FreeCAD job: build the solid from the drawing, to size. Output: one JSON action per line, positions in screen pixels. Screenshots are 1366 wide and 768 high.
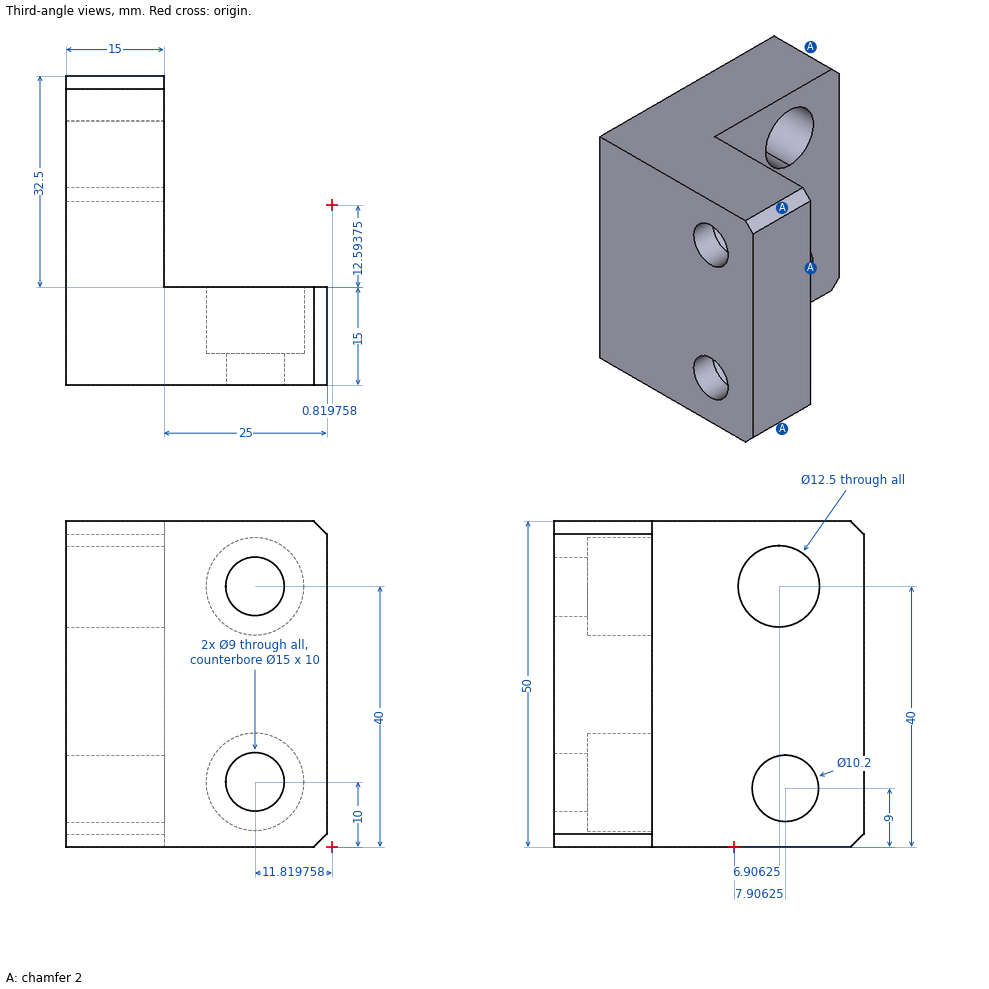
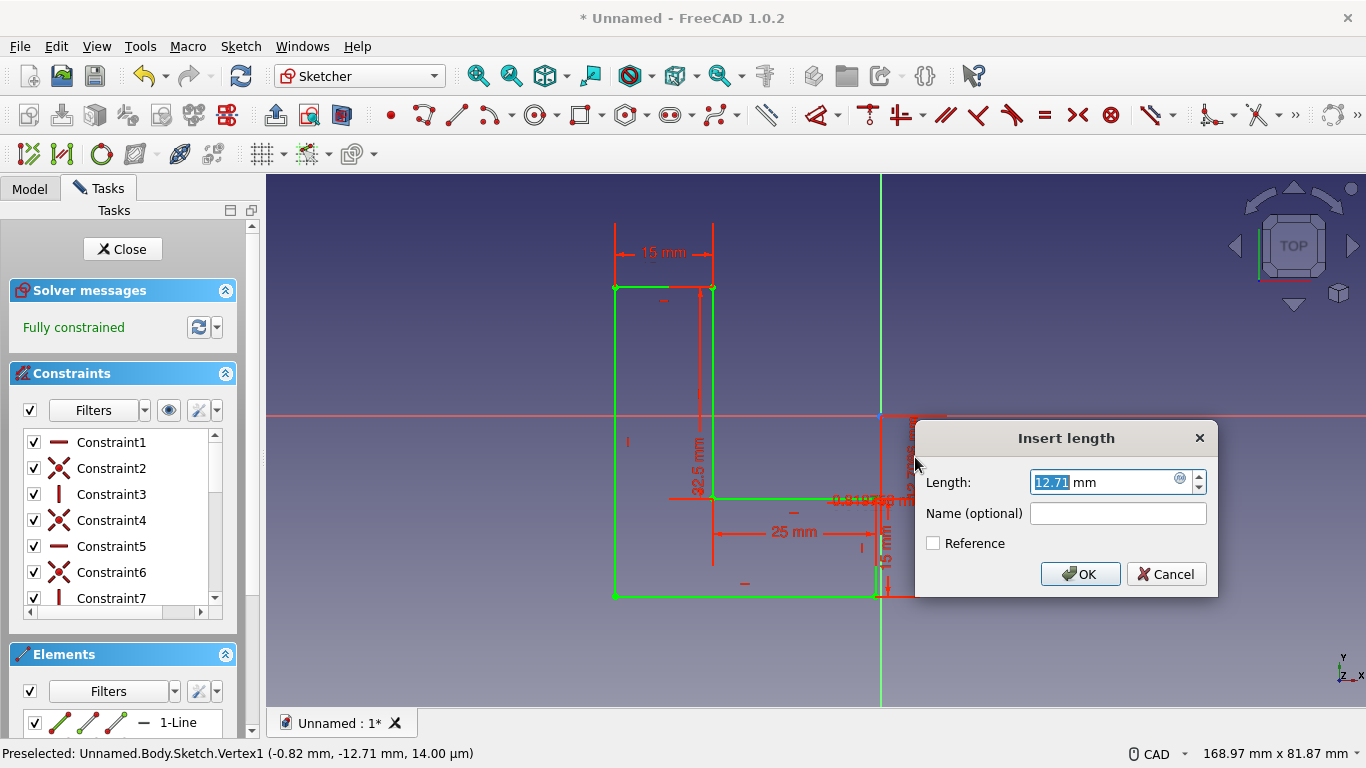
{"action": "type", "text": "12.59375"}
{"action": "key", "text": "Return"}
{"action": "key", "text": "Escape"}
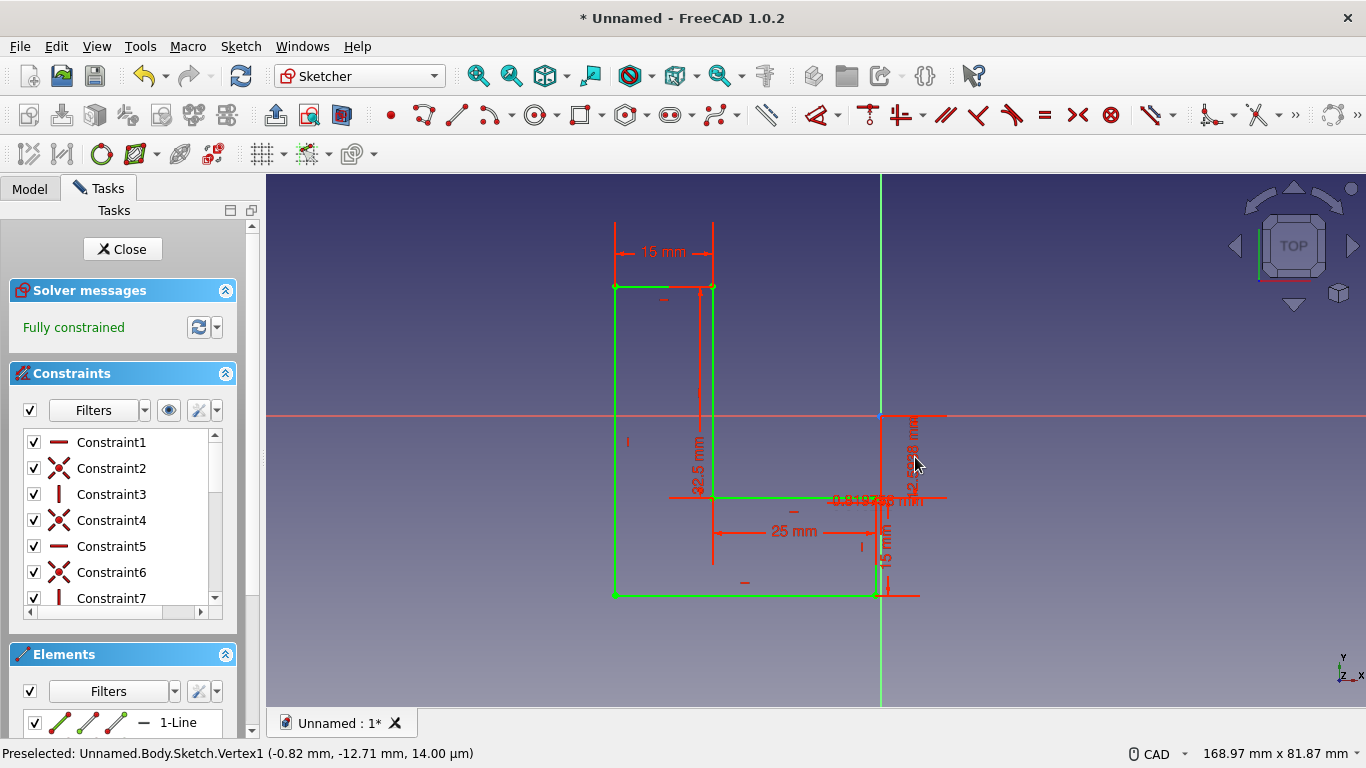
{"action": "left_click", "coordinate": [123, 249]}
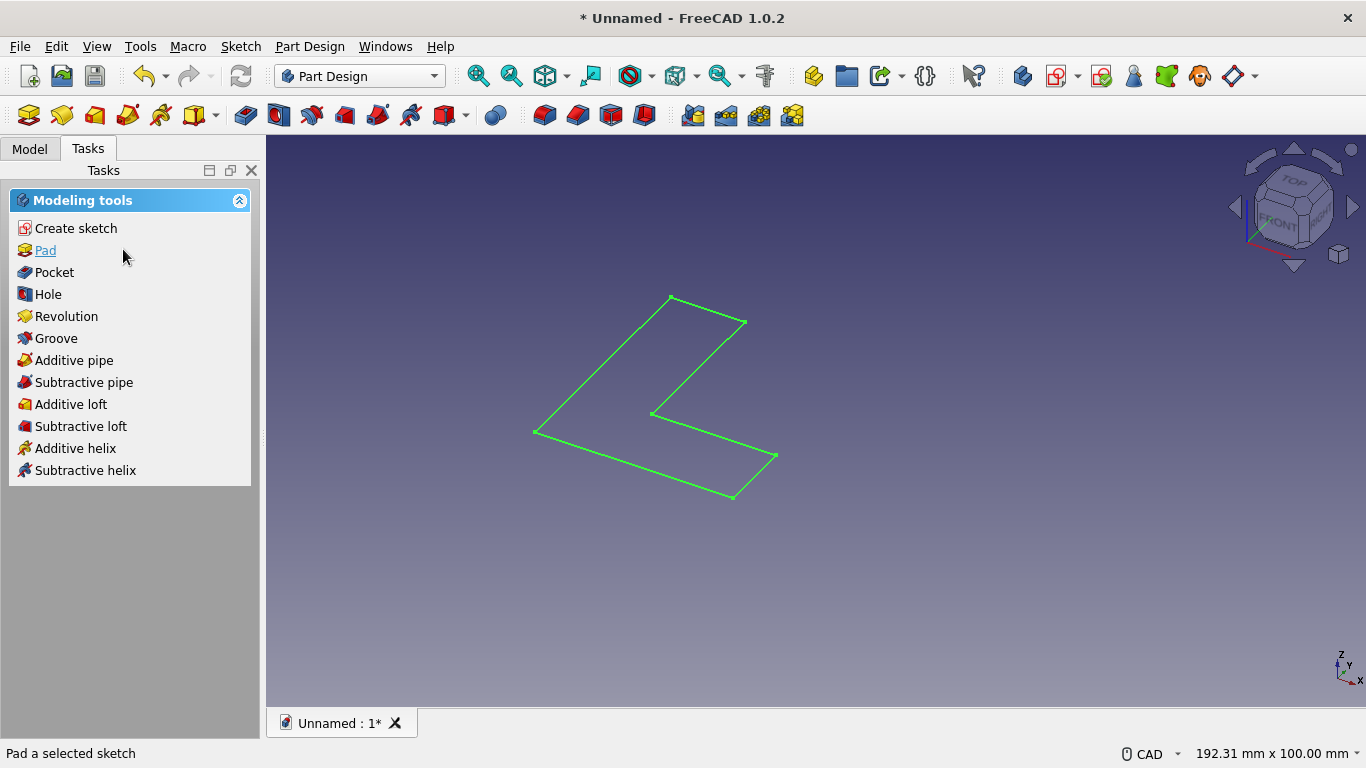
{"action": "left_click", "coordinate": [29, 116]}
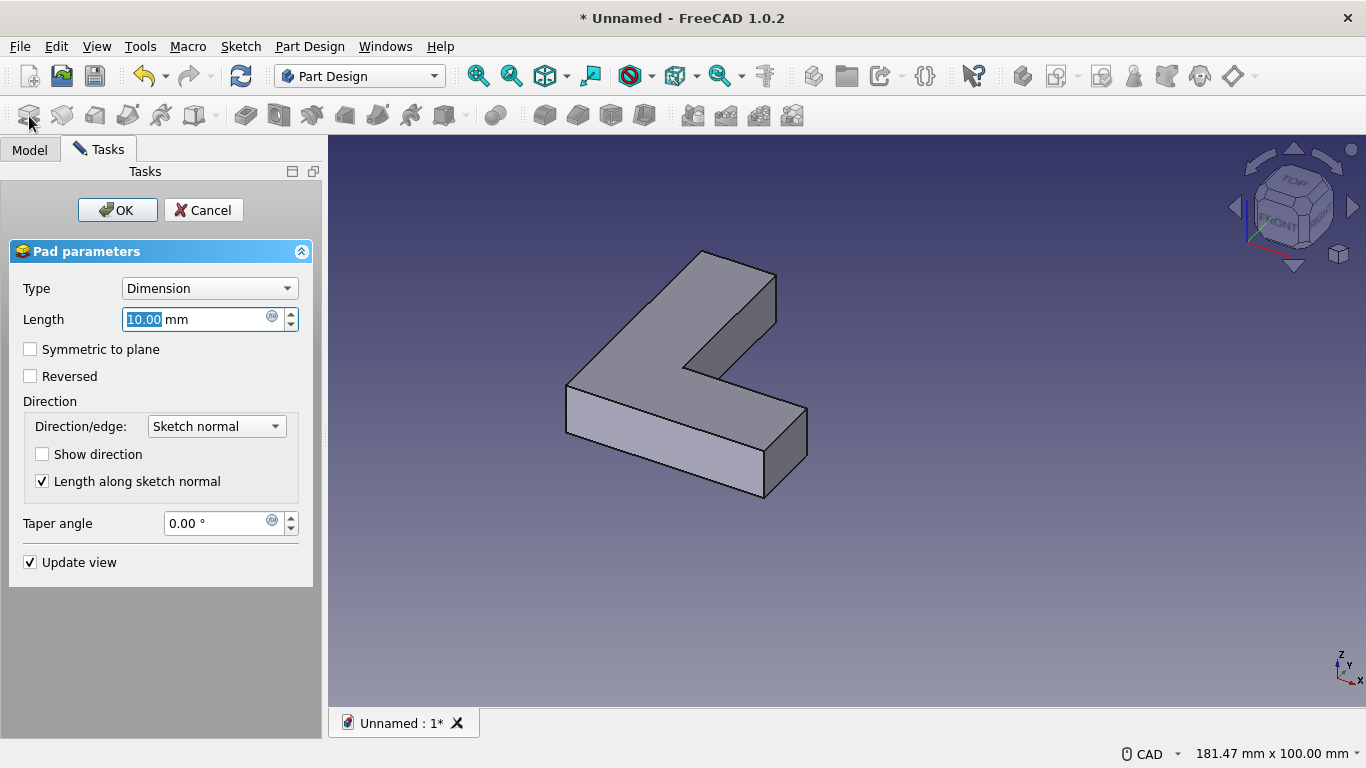
{"action": "type", "text": "50"}
{"action": "key", "text": "Tab"}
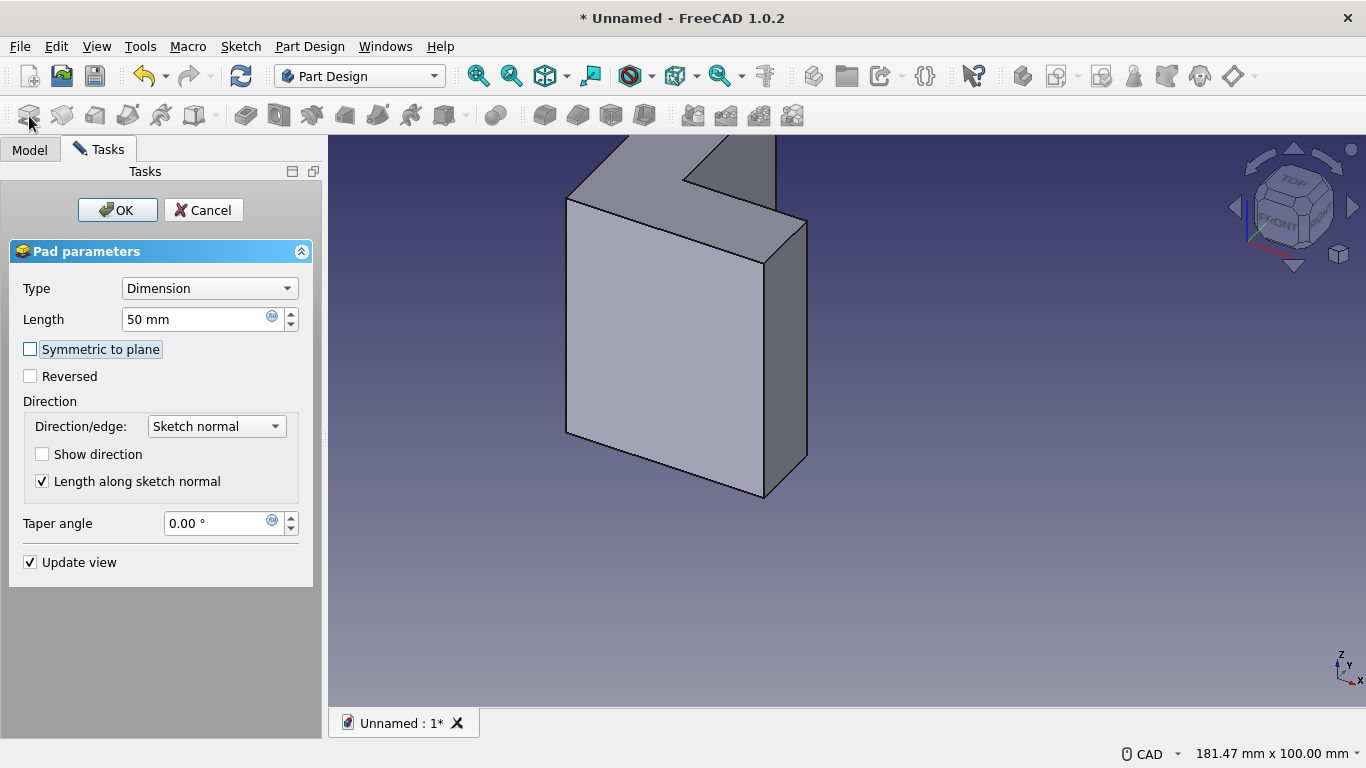
{"action": "left_click", "coordinate": [118, 210]}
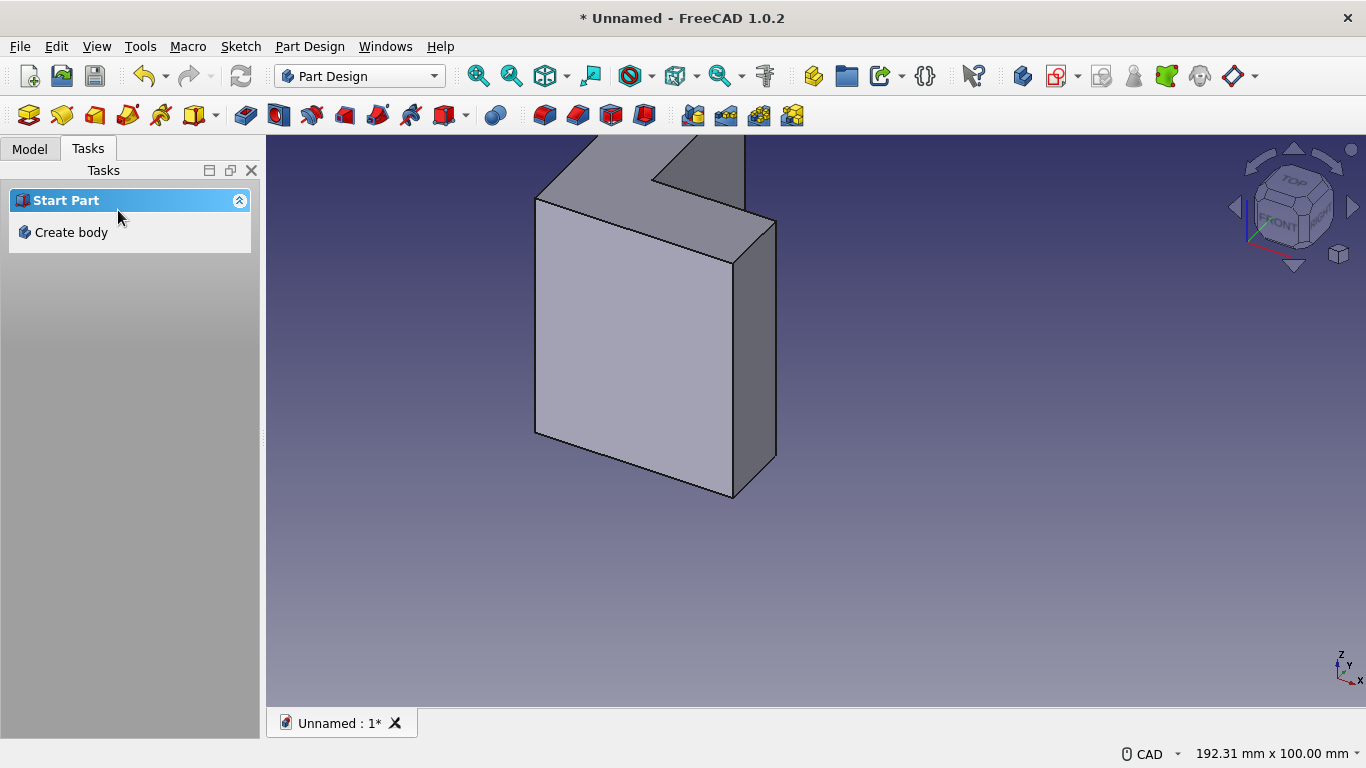
{"action": "left_click", "coordinate": [479, 76]}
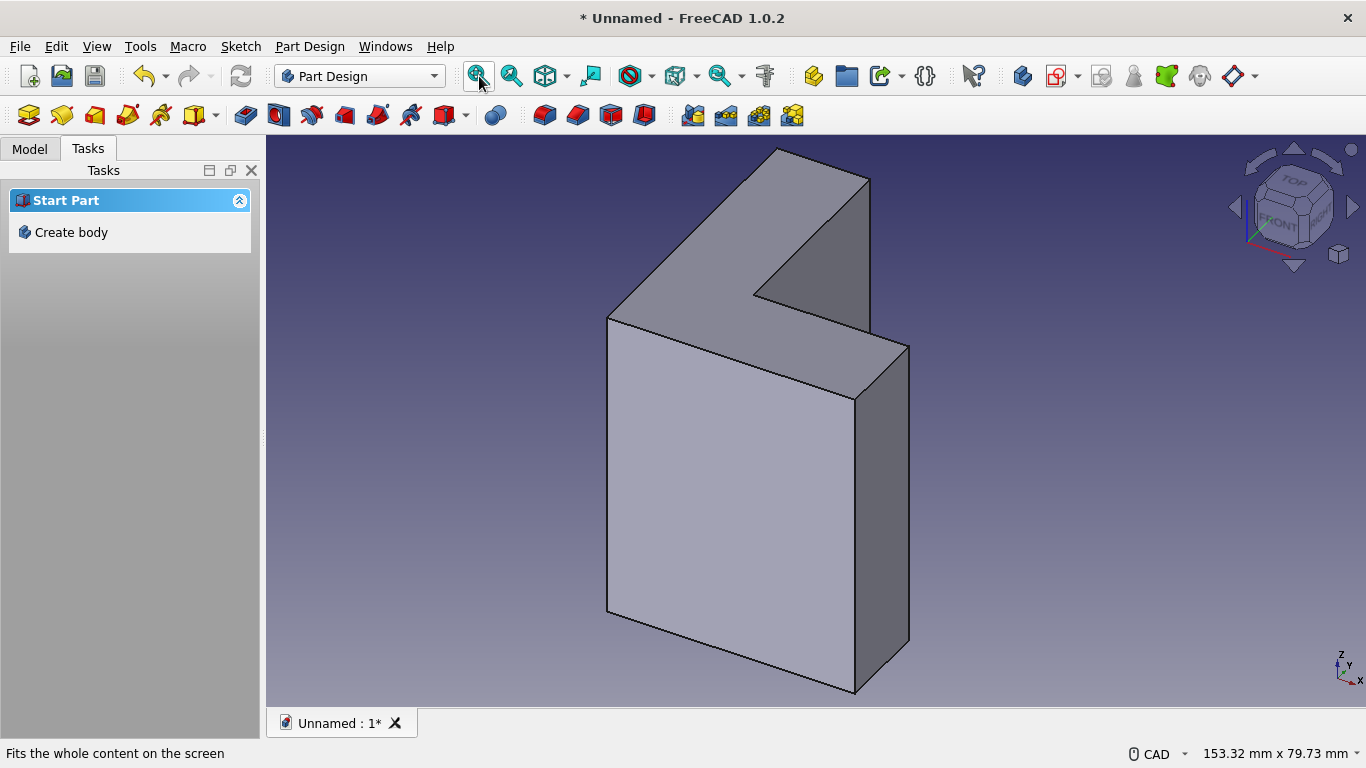
{"action": "left_click", "coordinate": [882, 372]}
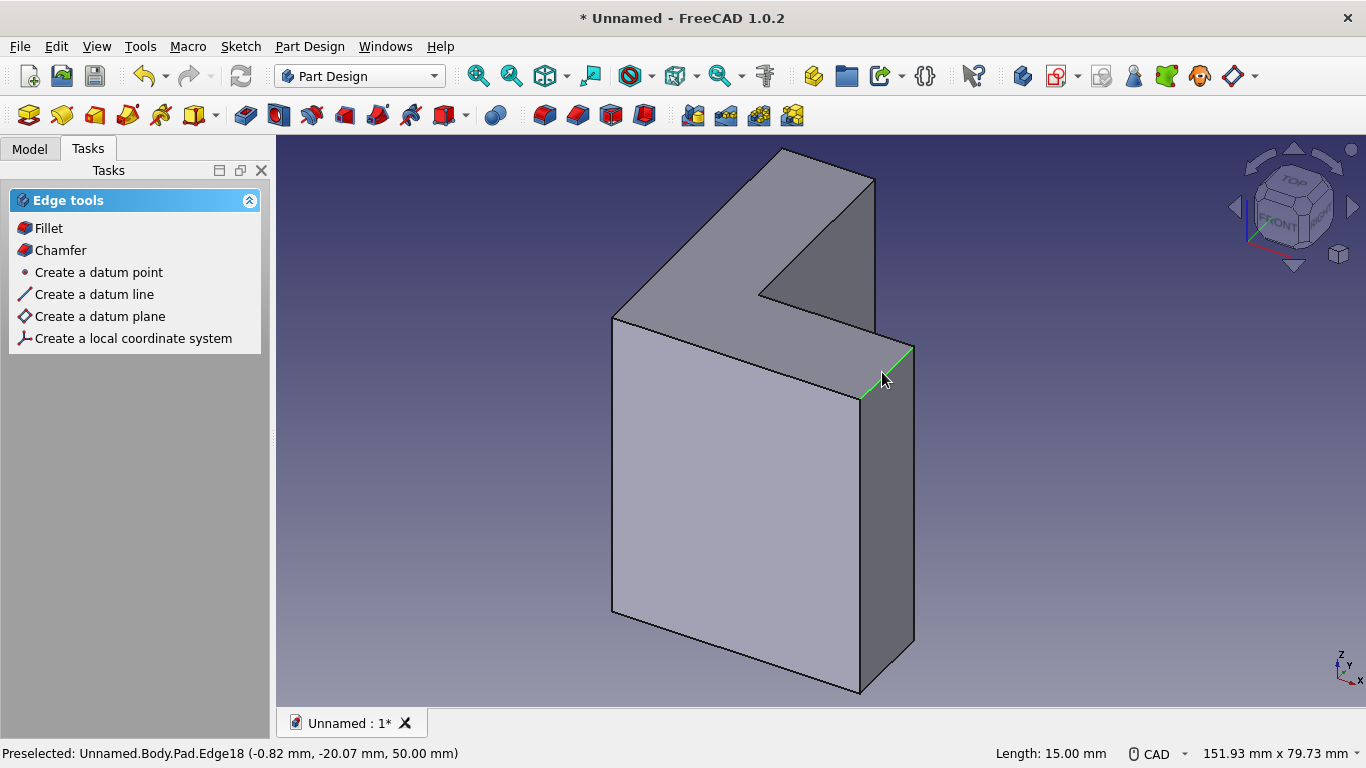
{"action": "key", "text": "0"}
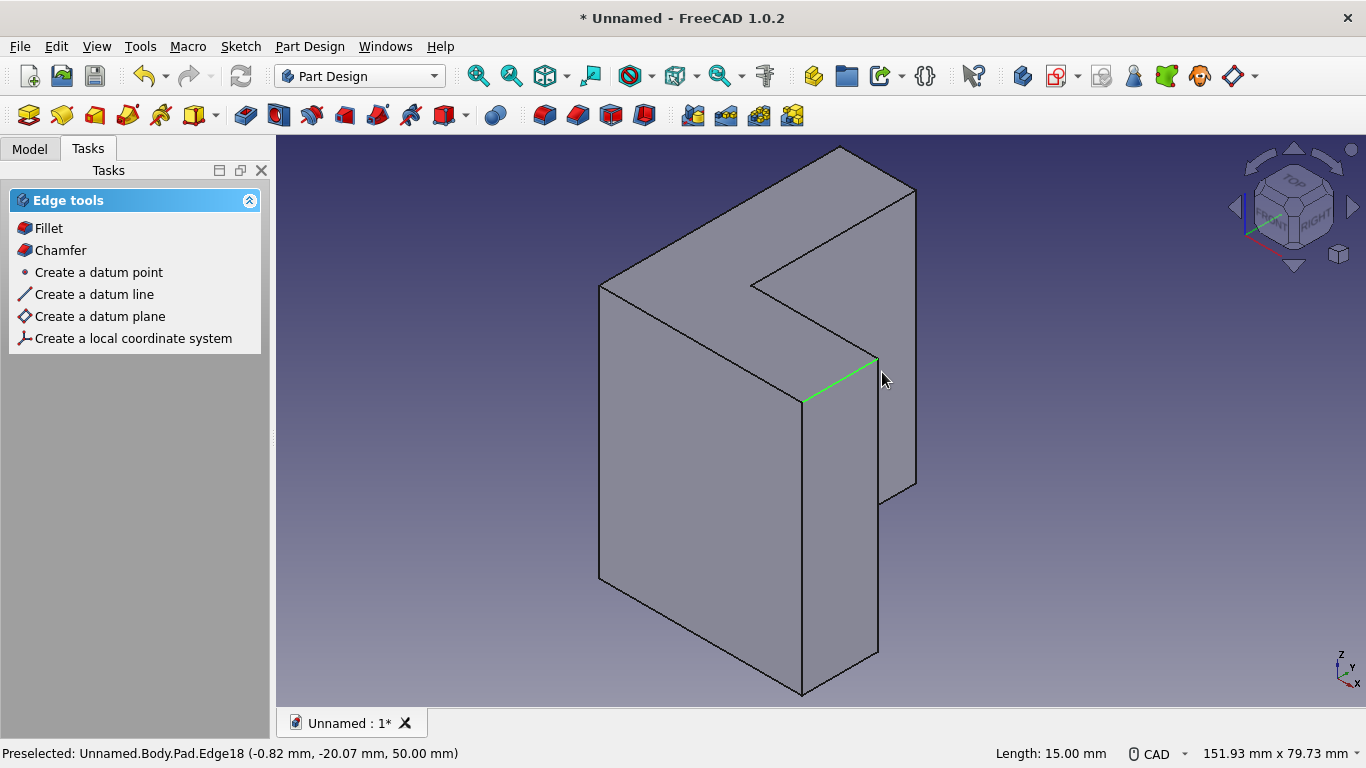
{"action": "key", "text": "2"}